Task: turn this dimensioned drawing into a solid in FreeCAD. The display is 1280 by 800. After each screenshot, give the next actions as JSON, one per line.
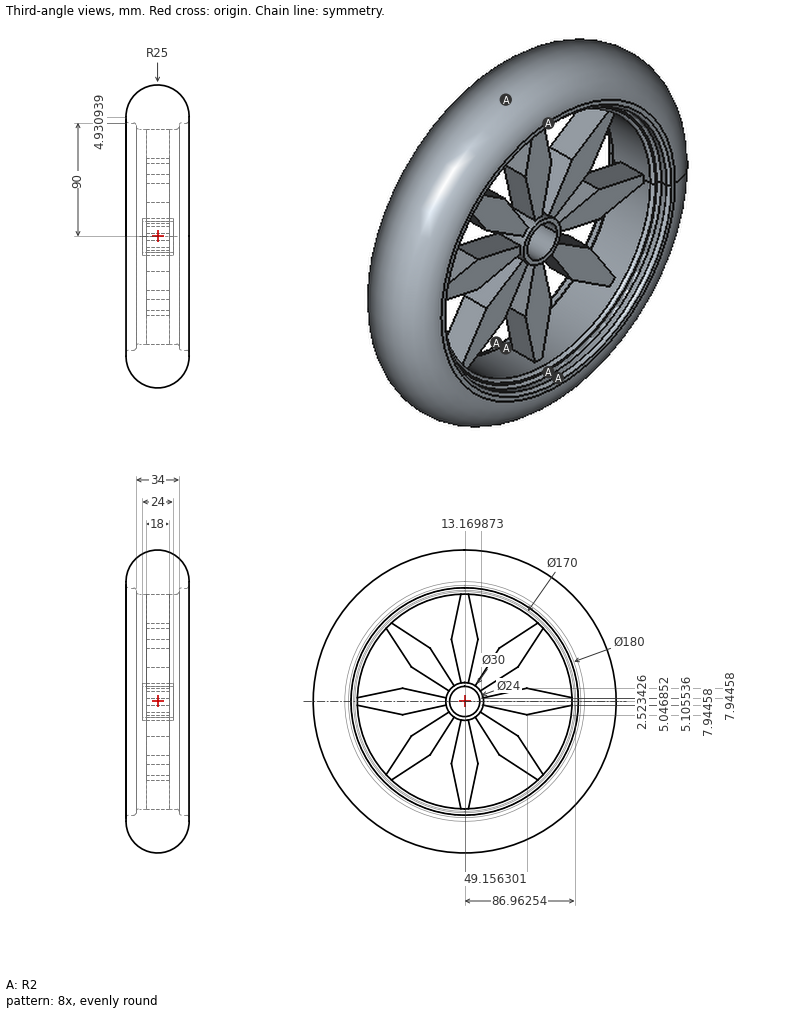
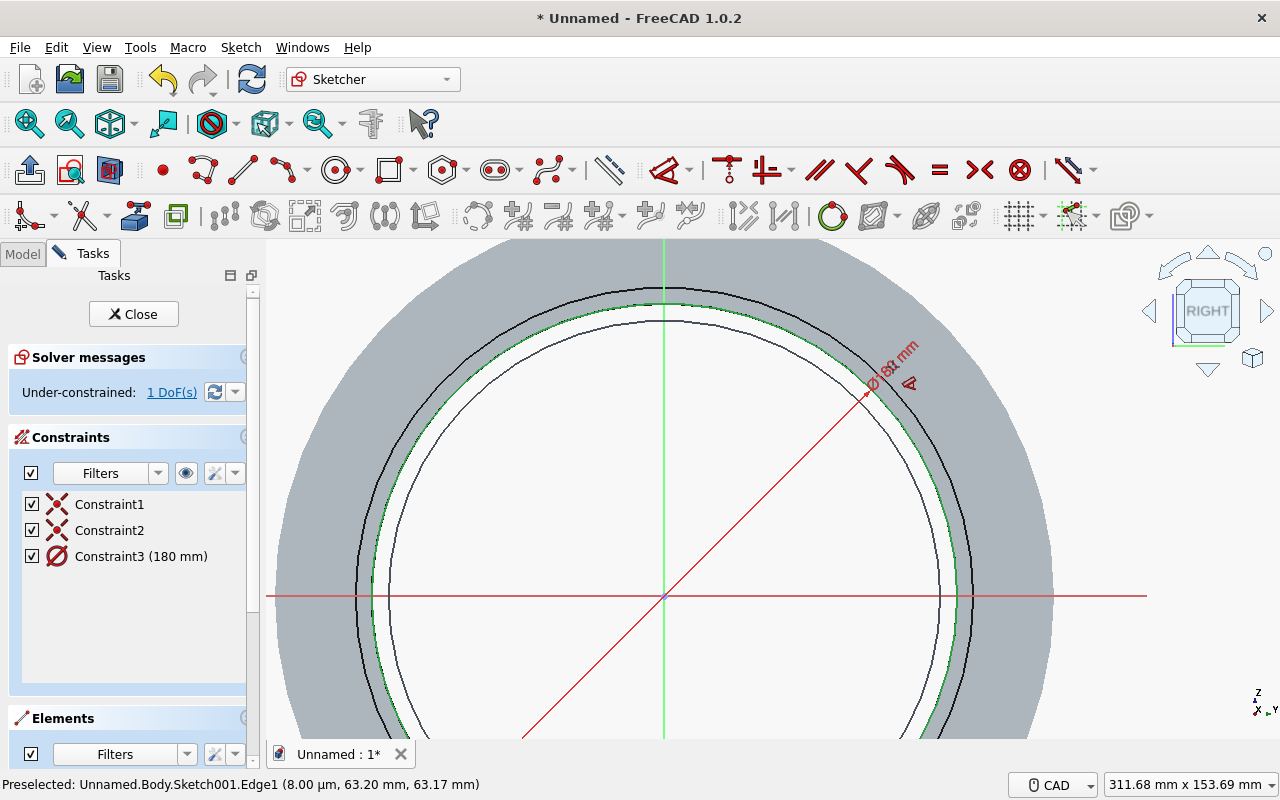
{"action": "left_click", "coordinate": [859, 401]}
{"action": "left_click", "coordinate": [960, 509]}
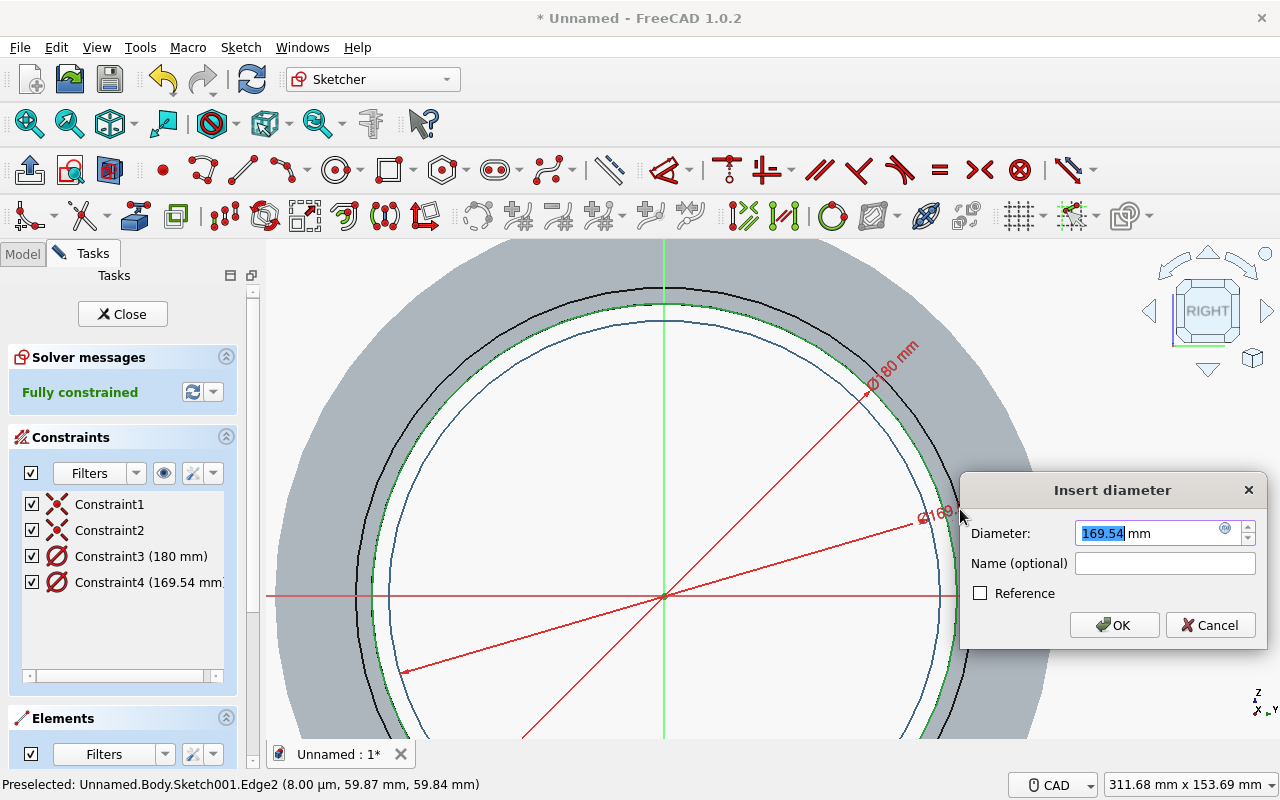
{"action": "type", "text": "170"}
{"action": "key", "text": "Return"}
{"action": "key", "text": "Escape"}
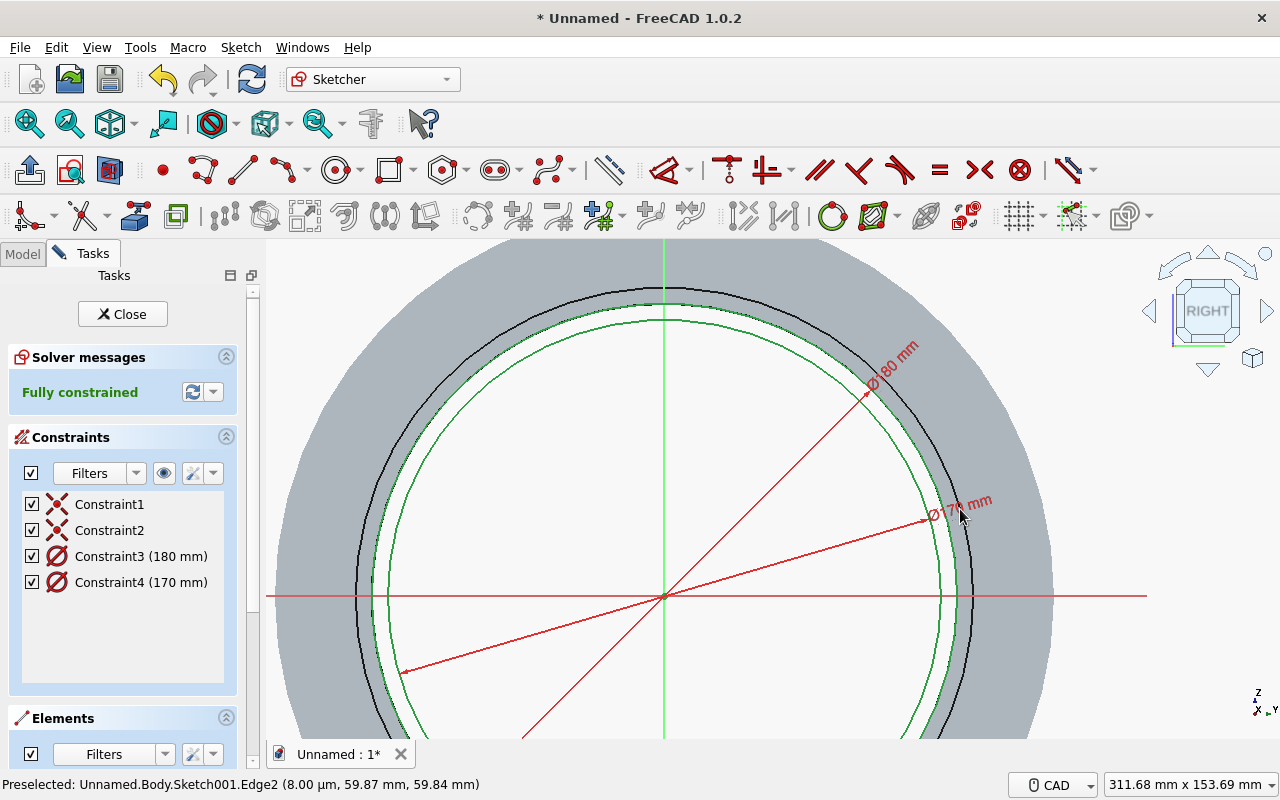
{"action": "left_click", "coordinate": [123, 314]}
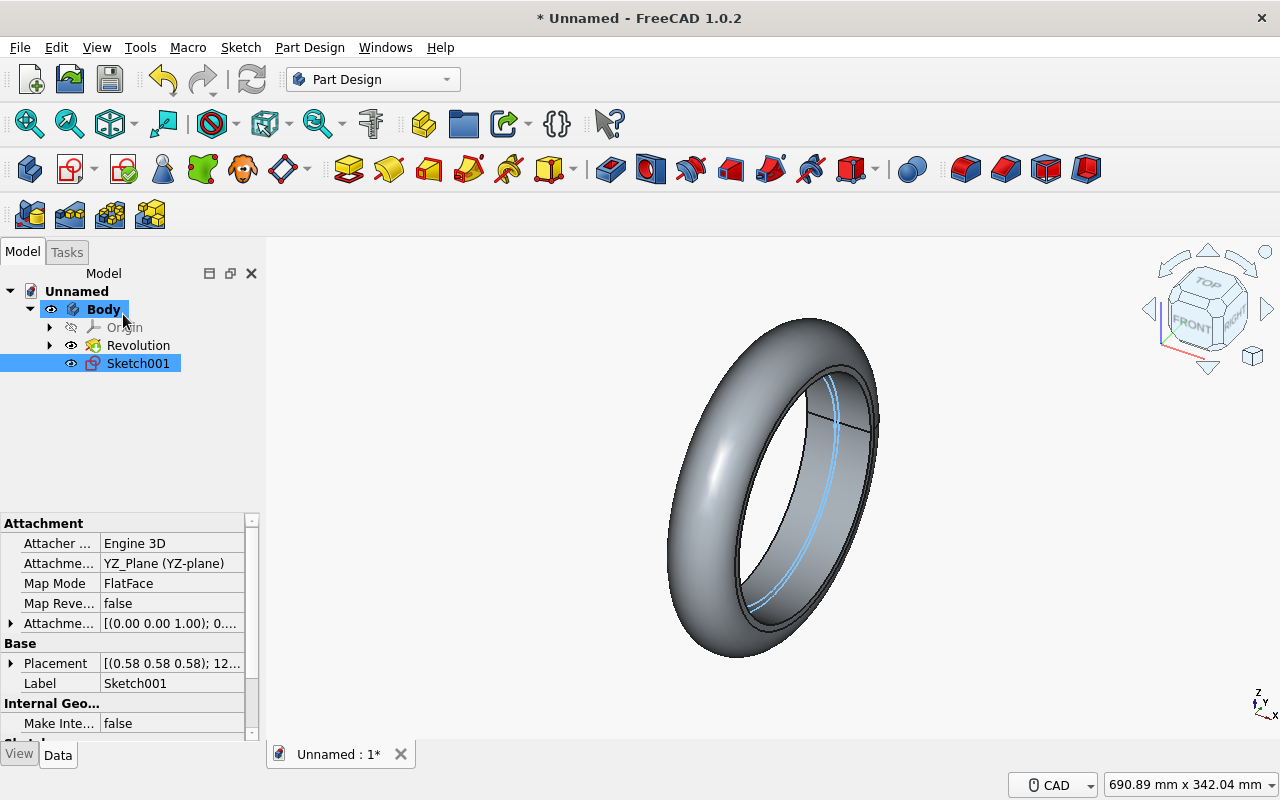
{"action": "left_click", "coordinate": [350, 170]}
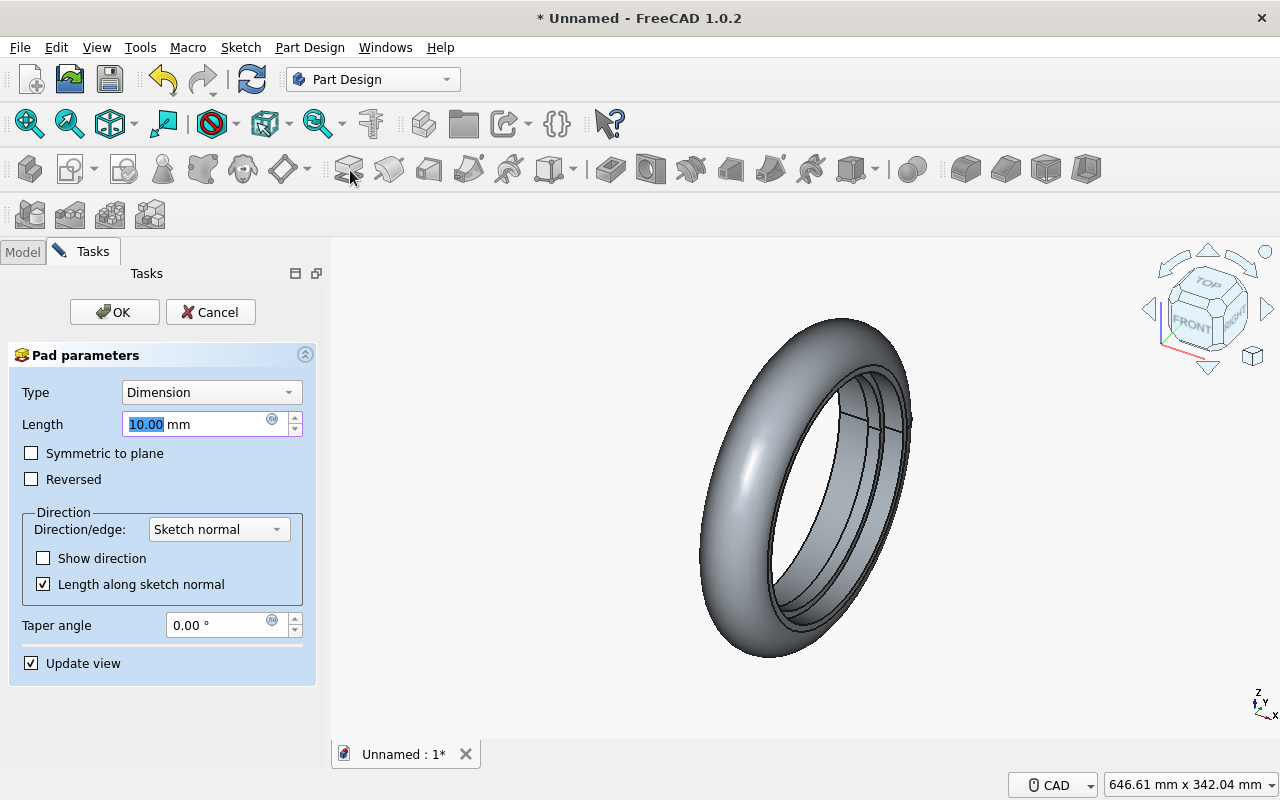
{"action": "type", "text": "34"}
{"action": "key", "text": "Tab"}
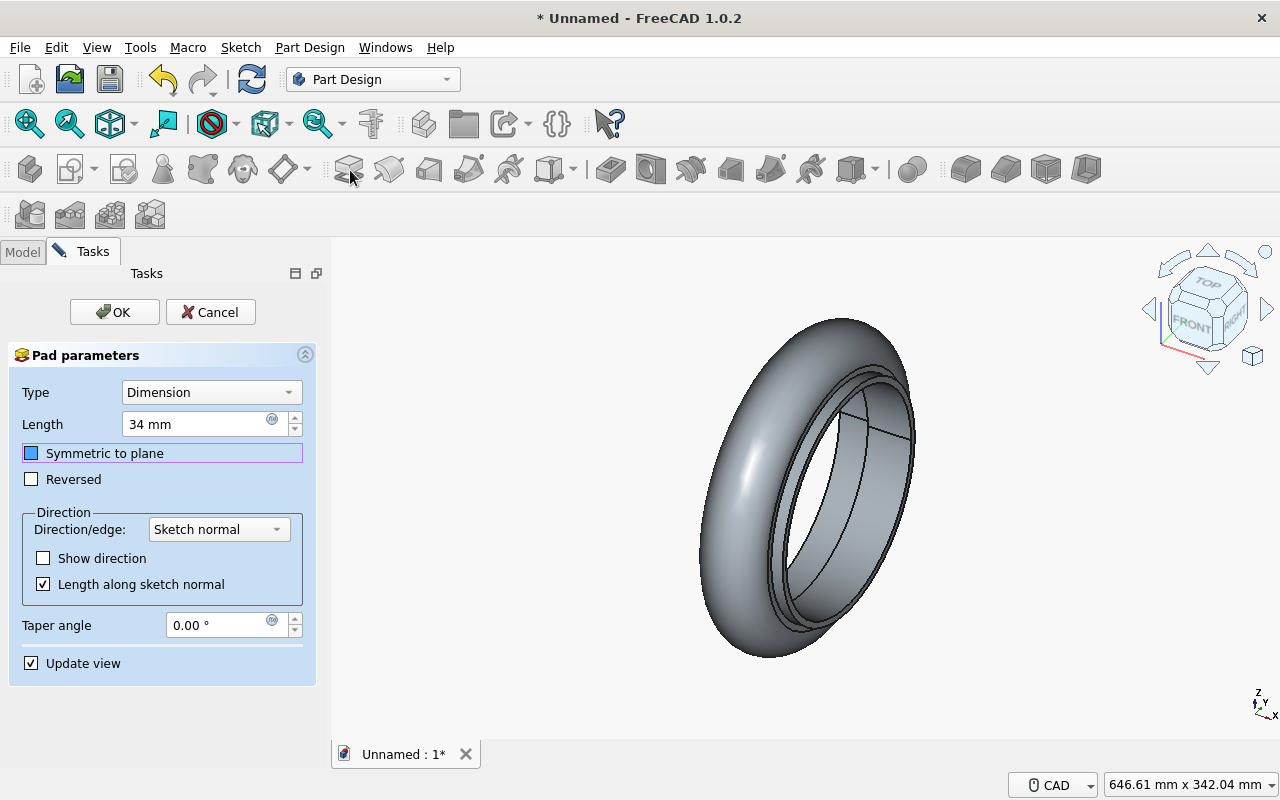
{"action": "left_click", "coordinate": [30, 453]}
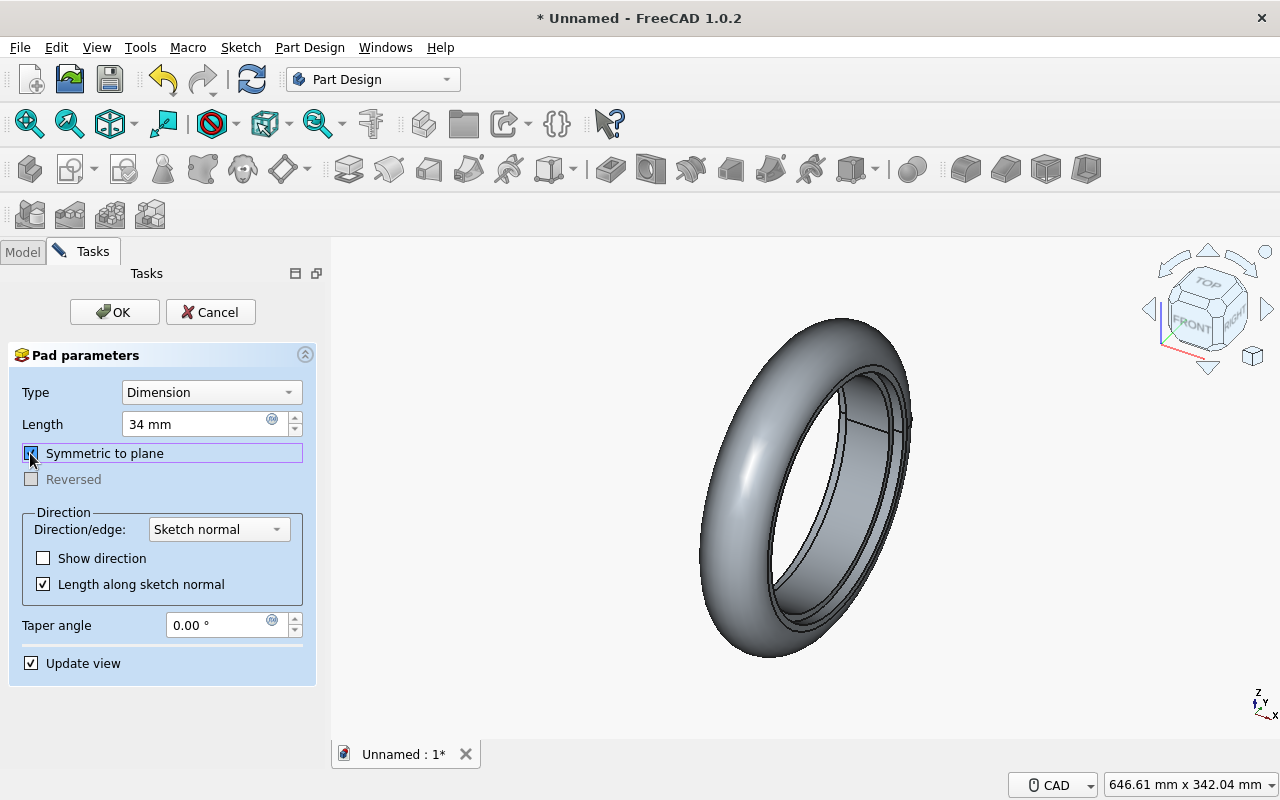
{"action": "left_click", "coordinate": [115, 312]}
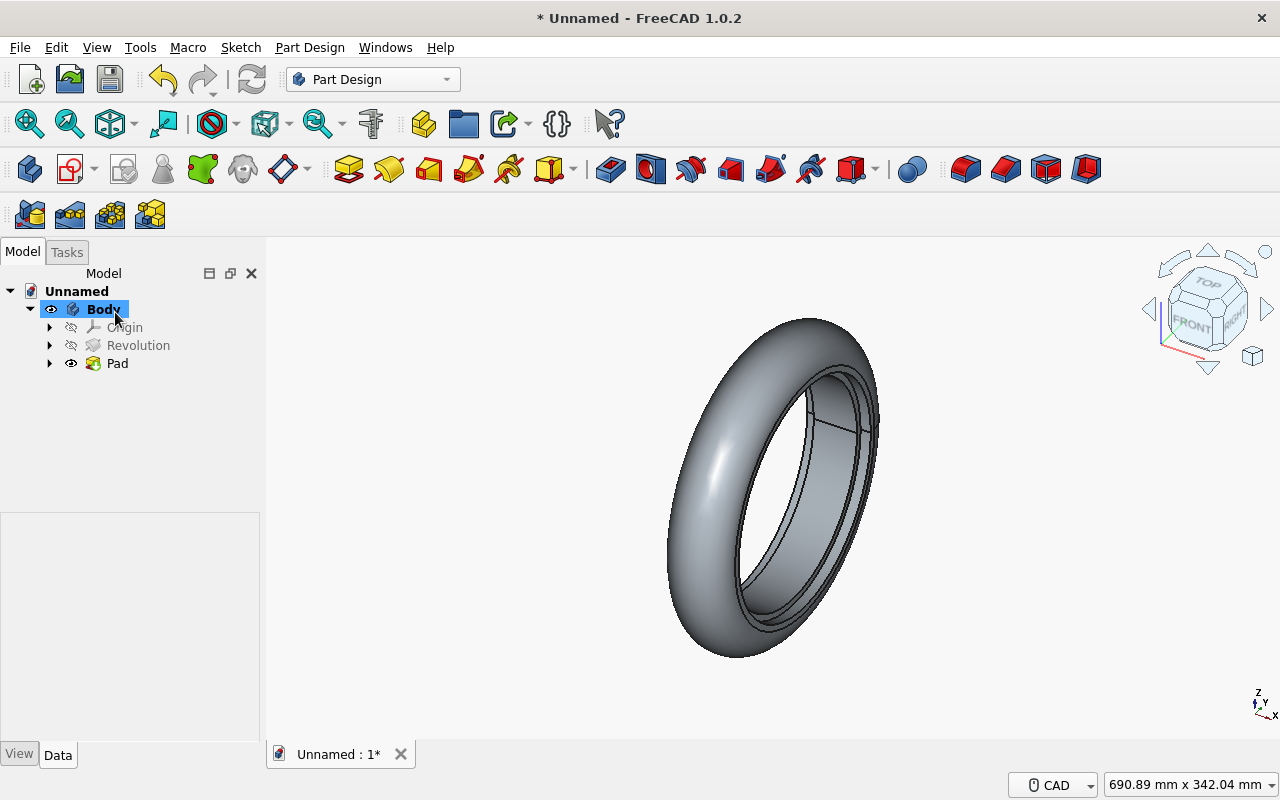
{"action": "left_click", "coordinate": [775, 610]}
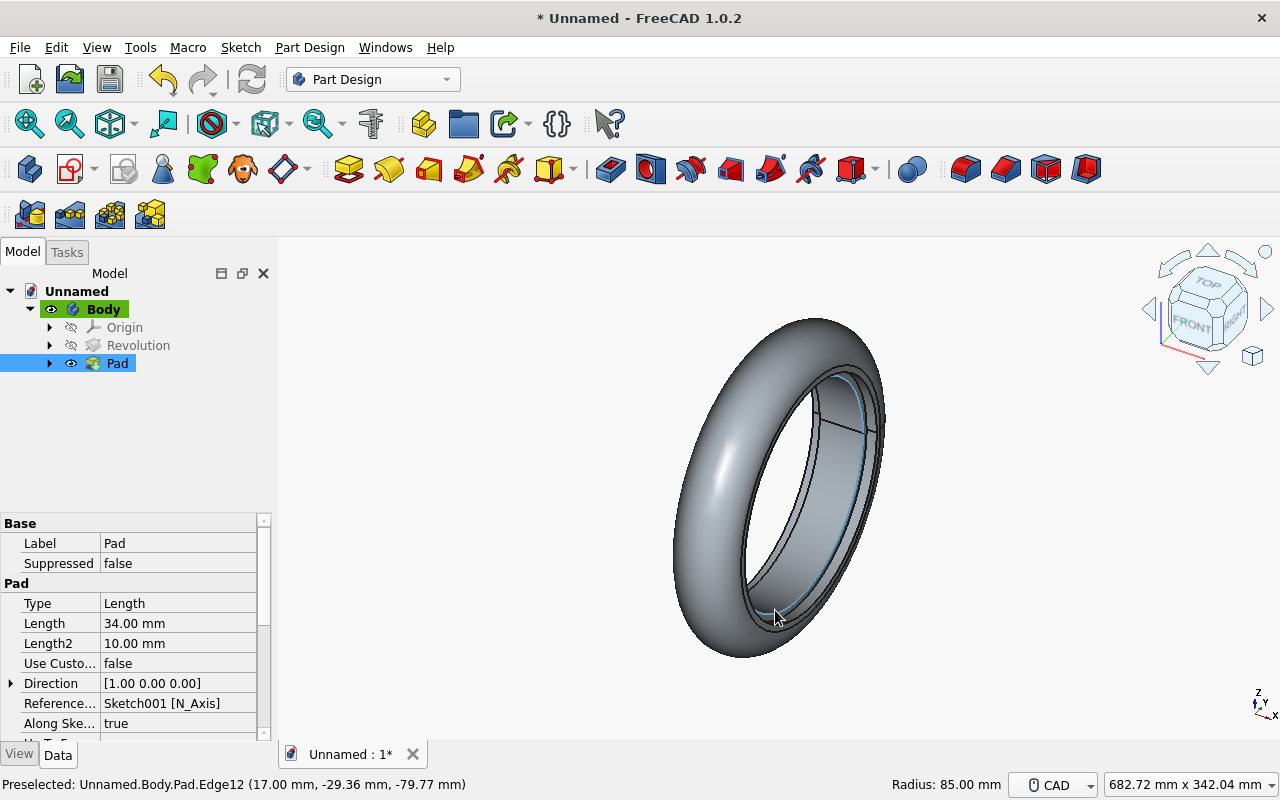
{"action": "left_click", "coordinate": [790, 621], "text": "ctrl"}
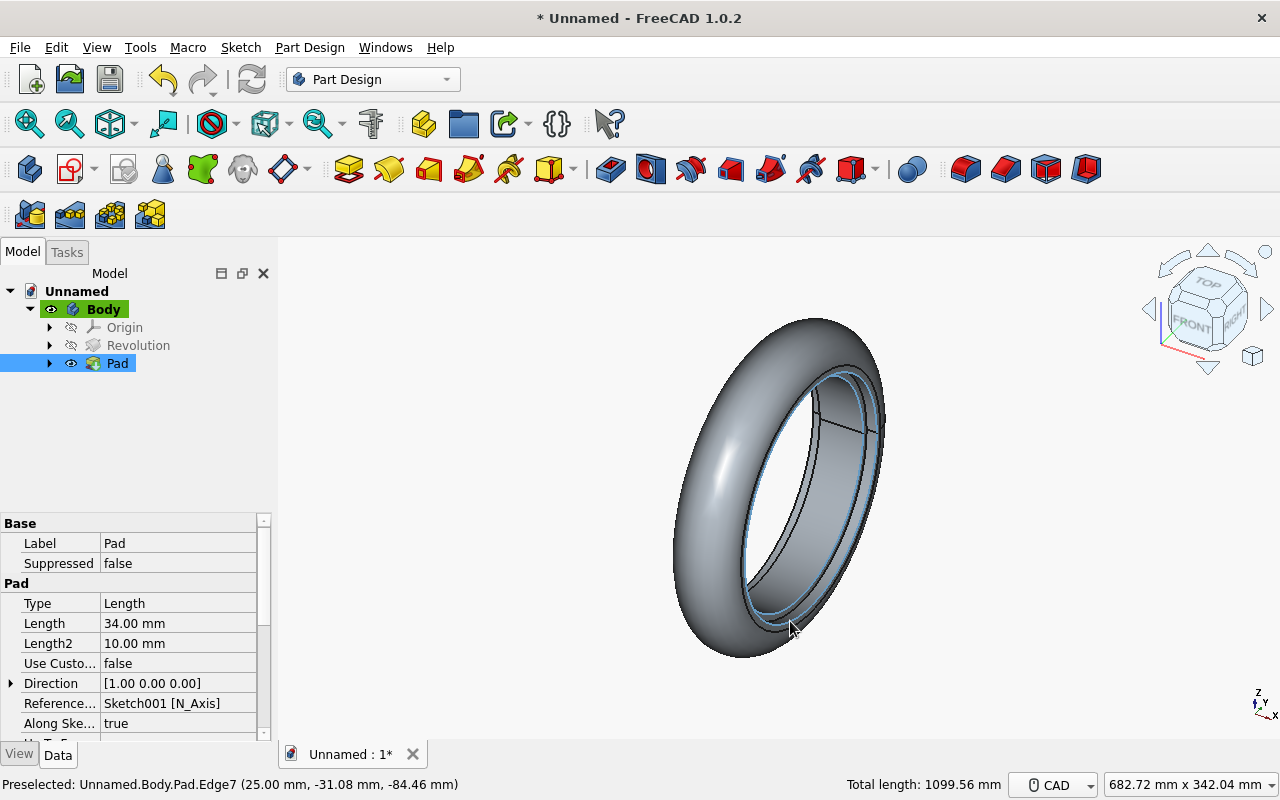
{"action": "key", "text": "0"}